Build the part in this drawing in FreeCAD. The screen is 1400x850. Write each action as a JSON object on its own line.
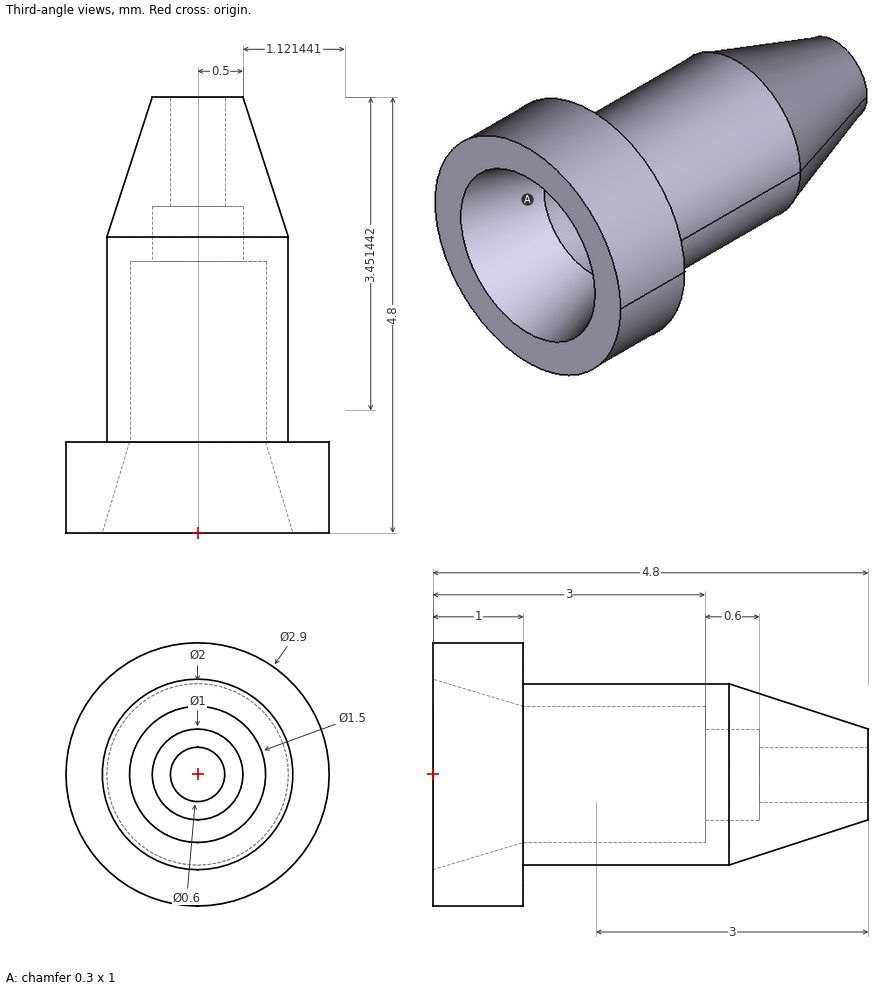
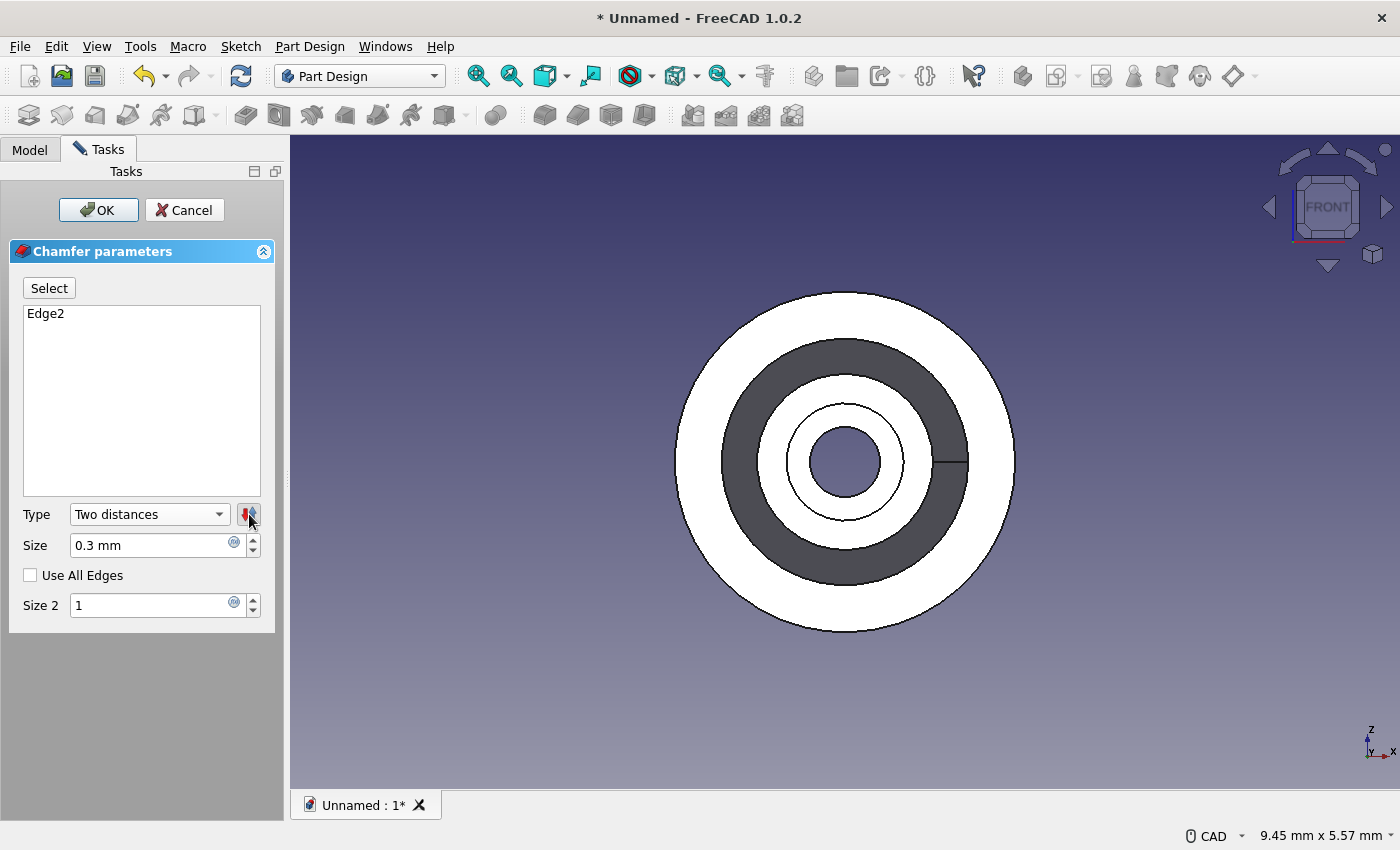
{"action": "left_click", "coordinate": [99, 210]}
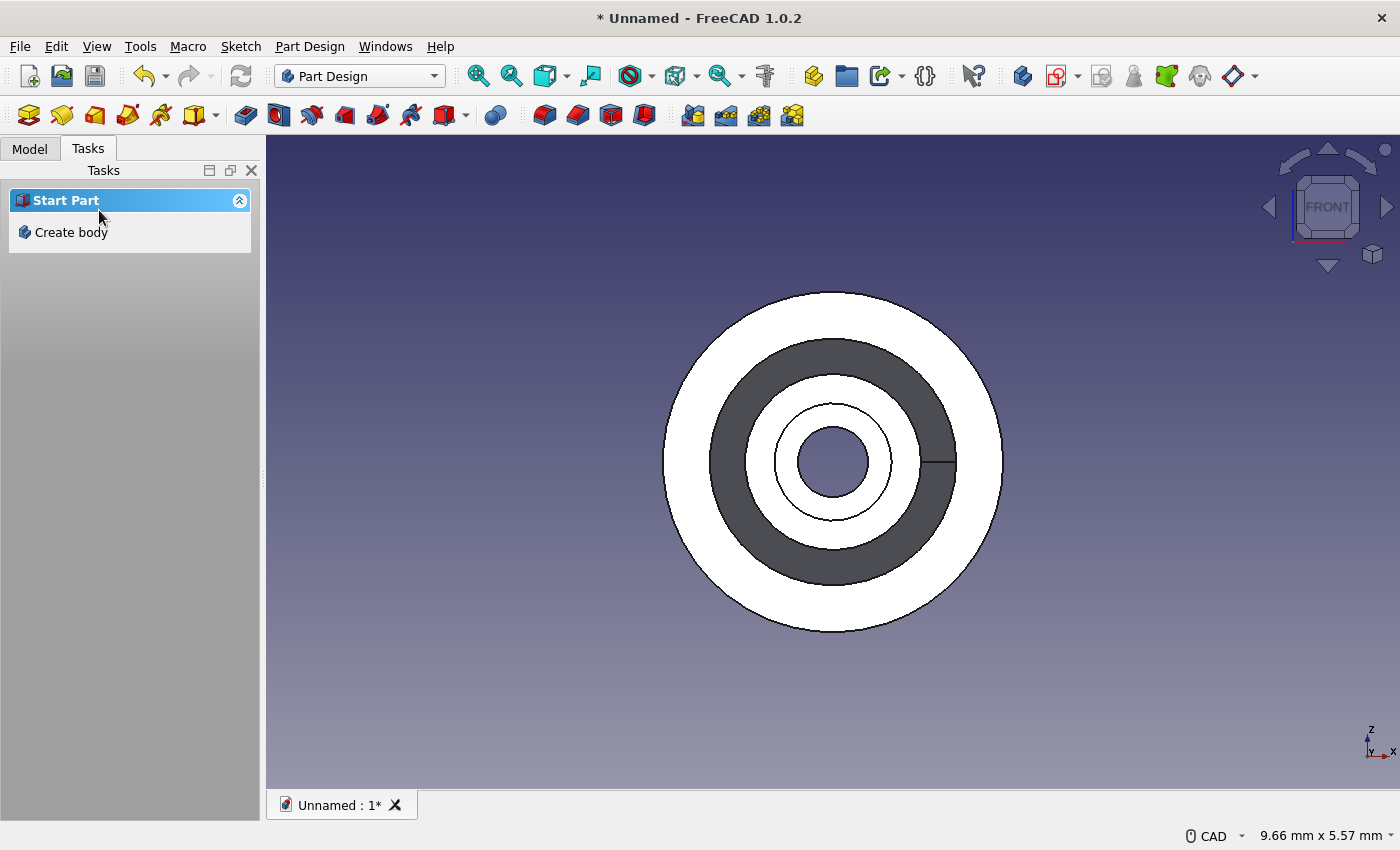
{"action": "key", "text": "0"}